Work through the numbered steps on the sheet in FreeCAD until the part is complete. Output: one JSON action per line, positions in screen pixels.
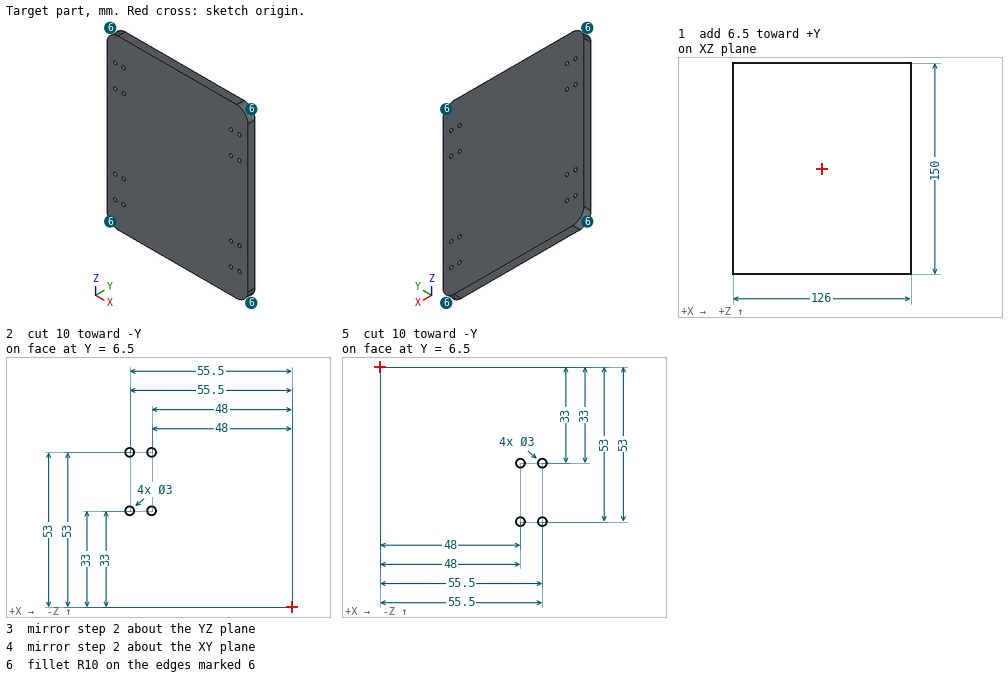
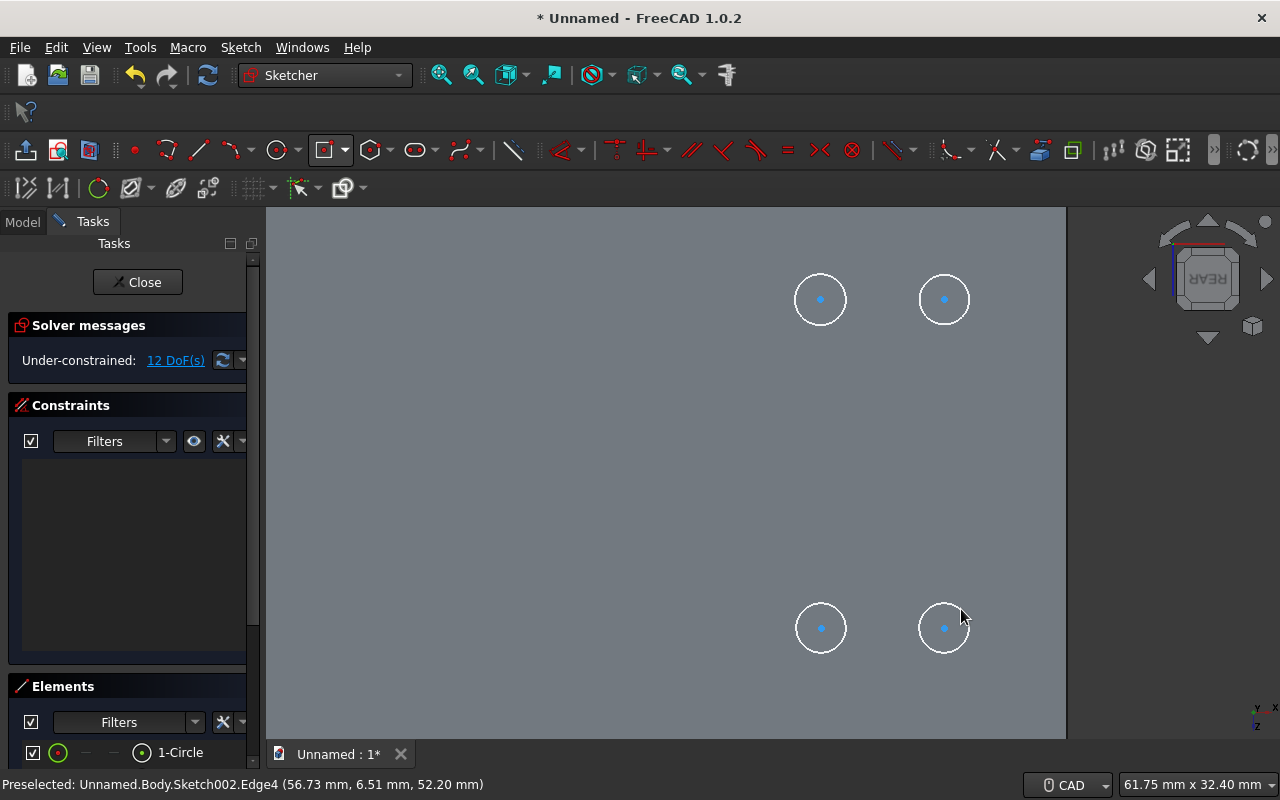
{"action": "left_click", "coordinate": [962, 282]}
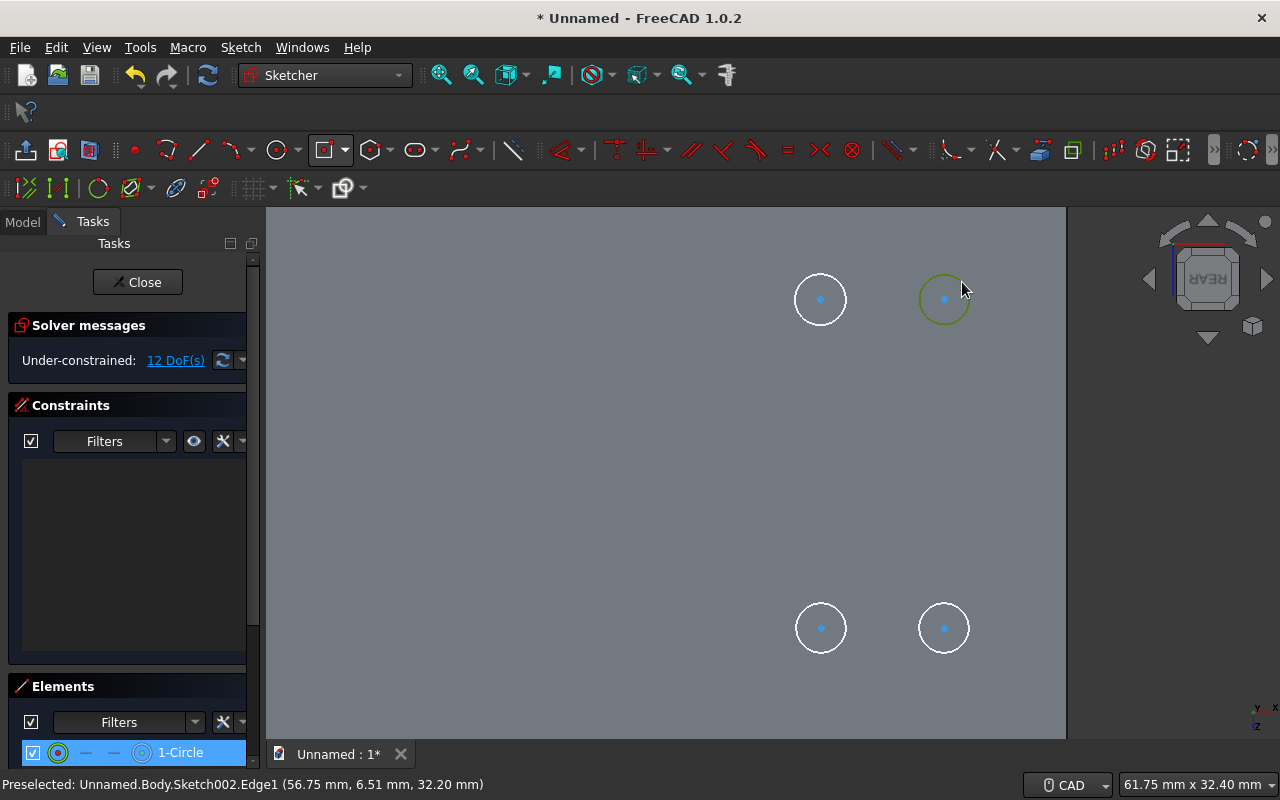
{"action": "left_click", "coordinate": [838, 282]}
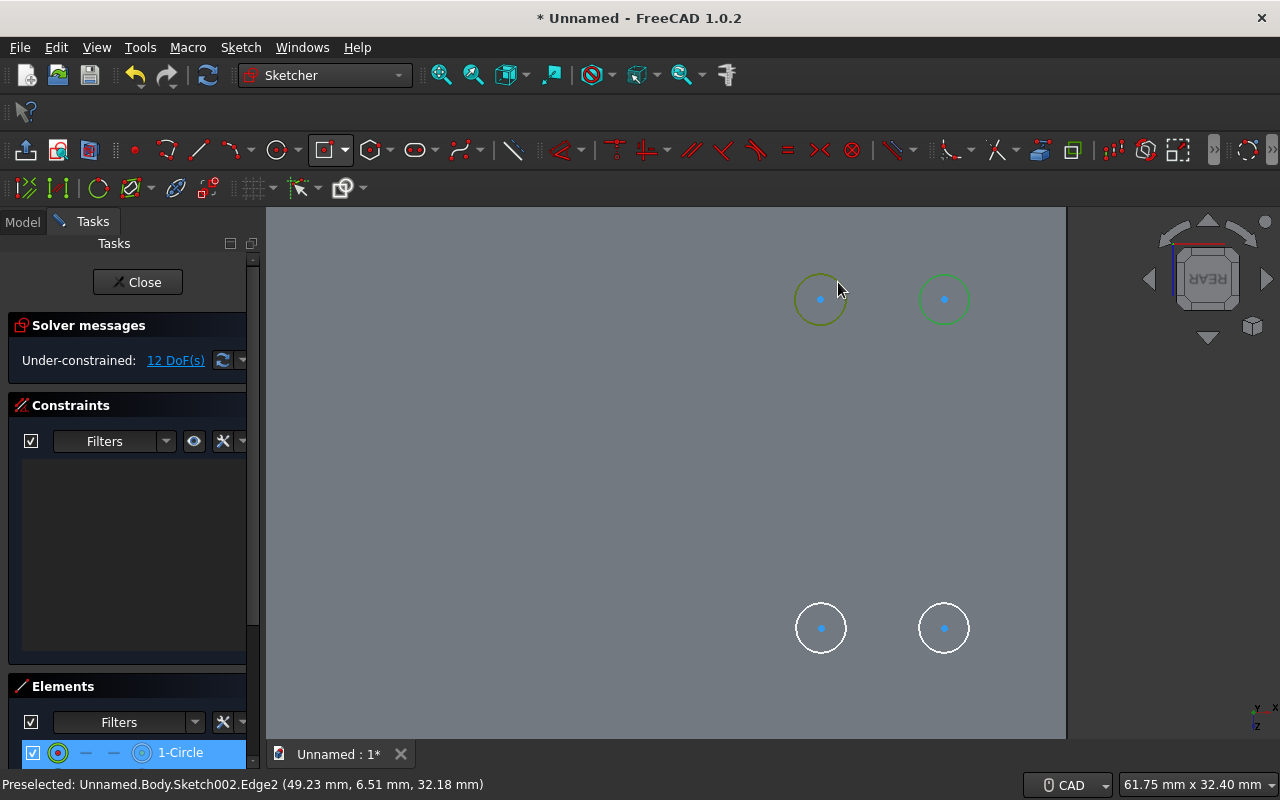
{"action": "left_click", "coordinate": [838, 610]}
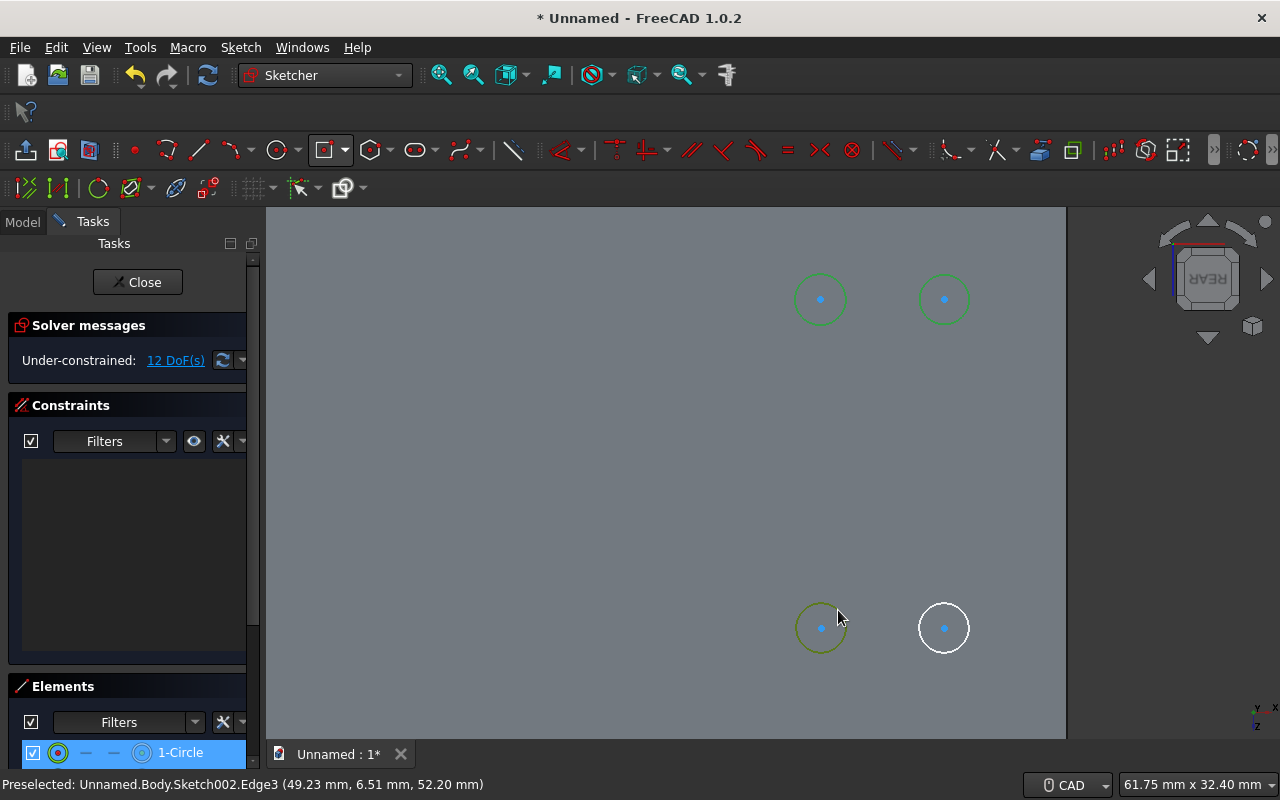
{"action": "left_click", "coordinate": [961, 610]}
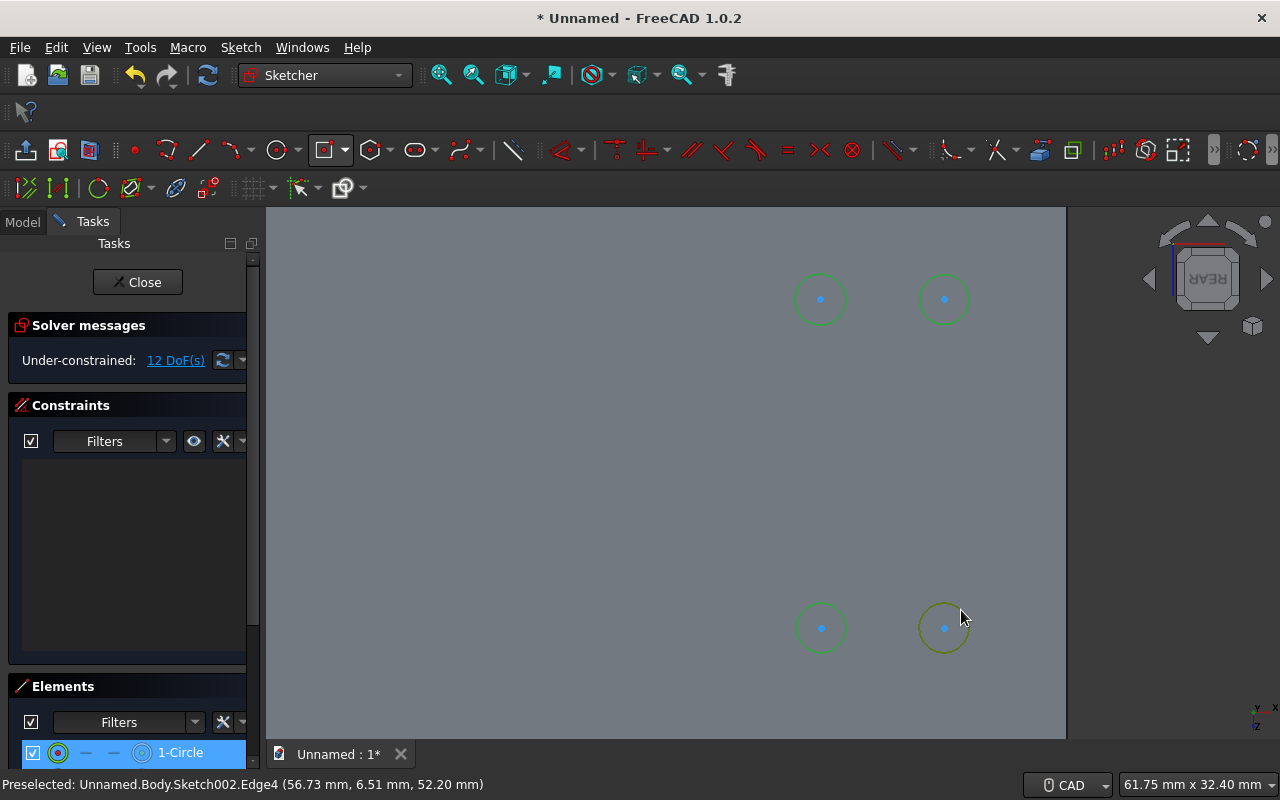
{"action": "left_click", "coordinate": [788, 150]}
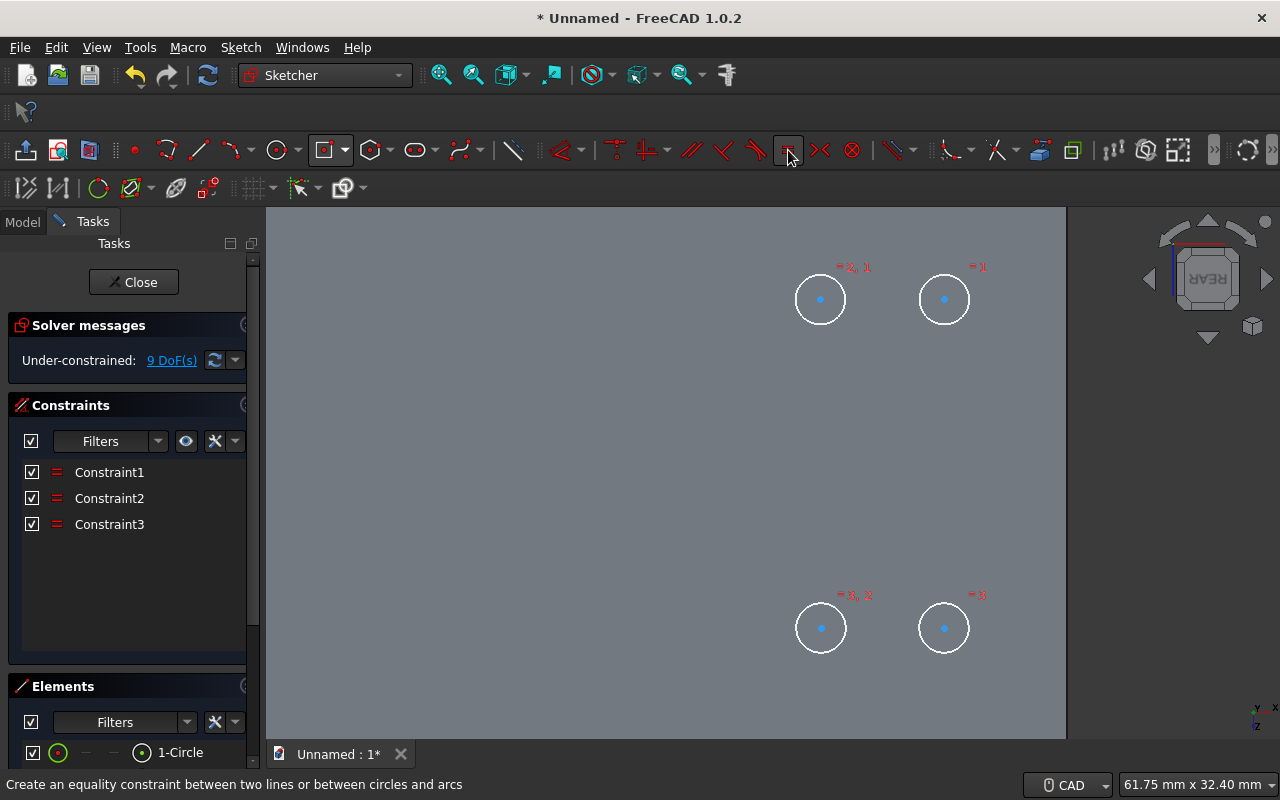
{"action": "left_click", "coordinate": [560, 150]}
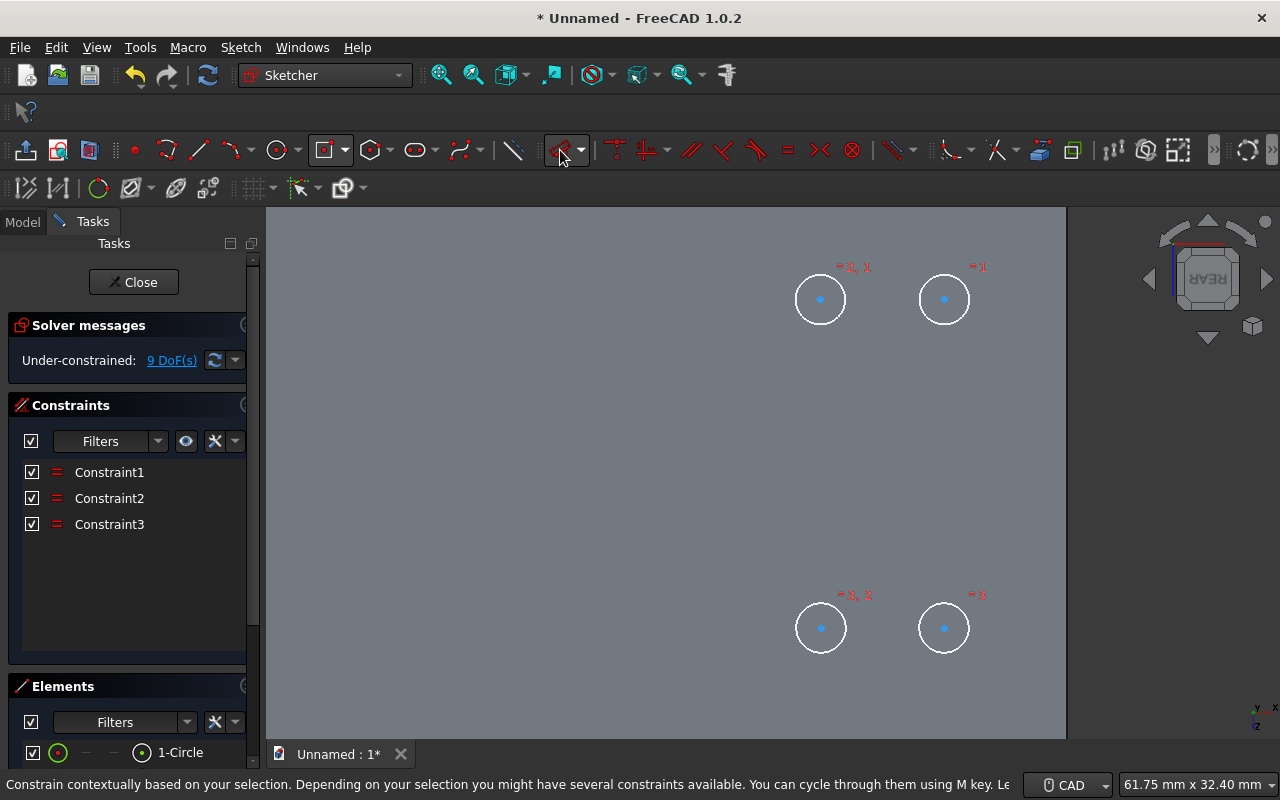
{"action": "left_click", "coordinate": [962, 282]}
{"action": "left_click", "coordinate": [985, 259]}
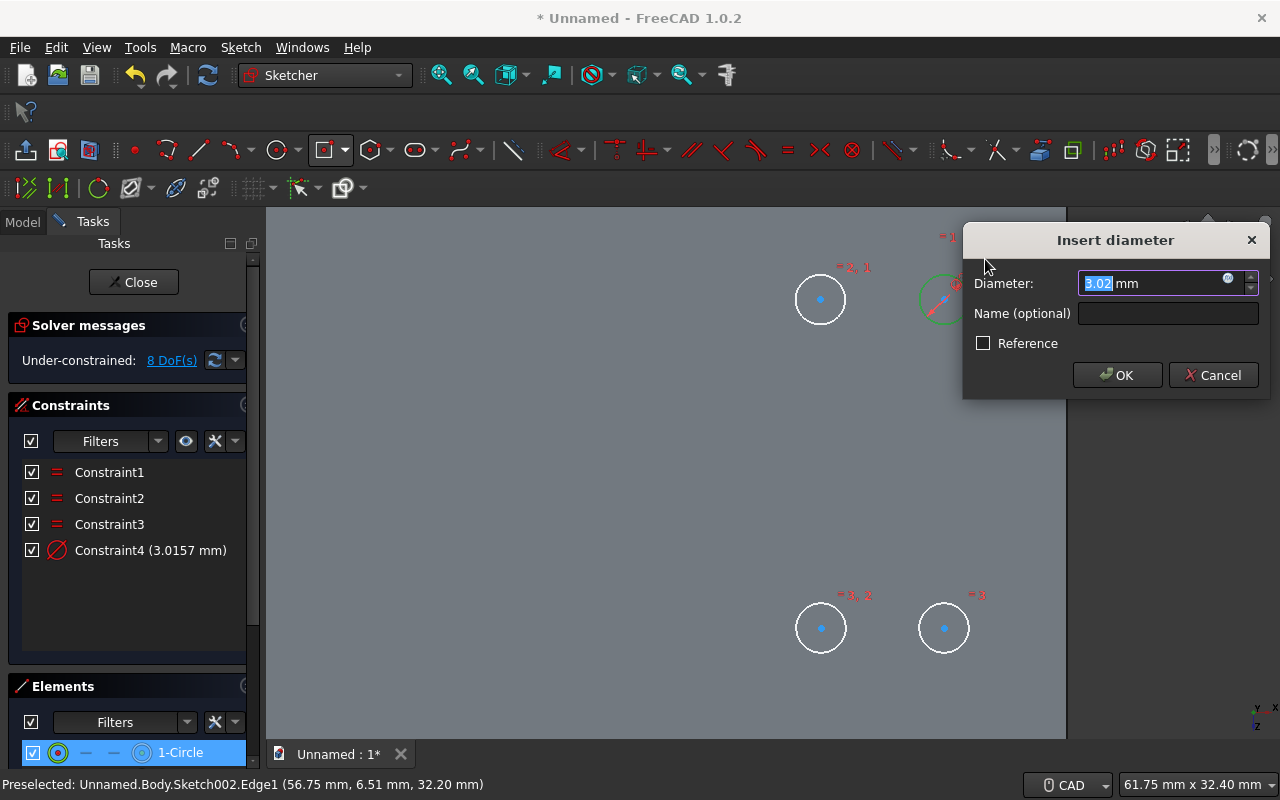
{"action": "type", "text": "3"}
{"action": "key", "text": "Return"}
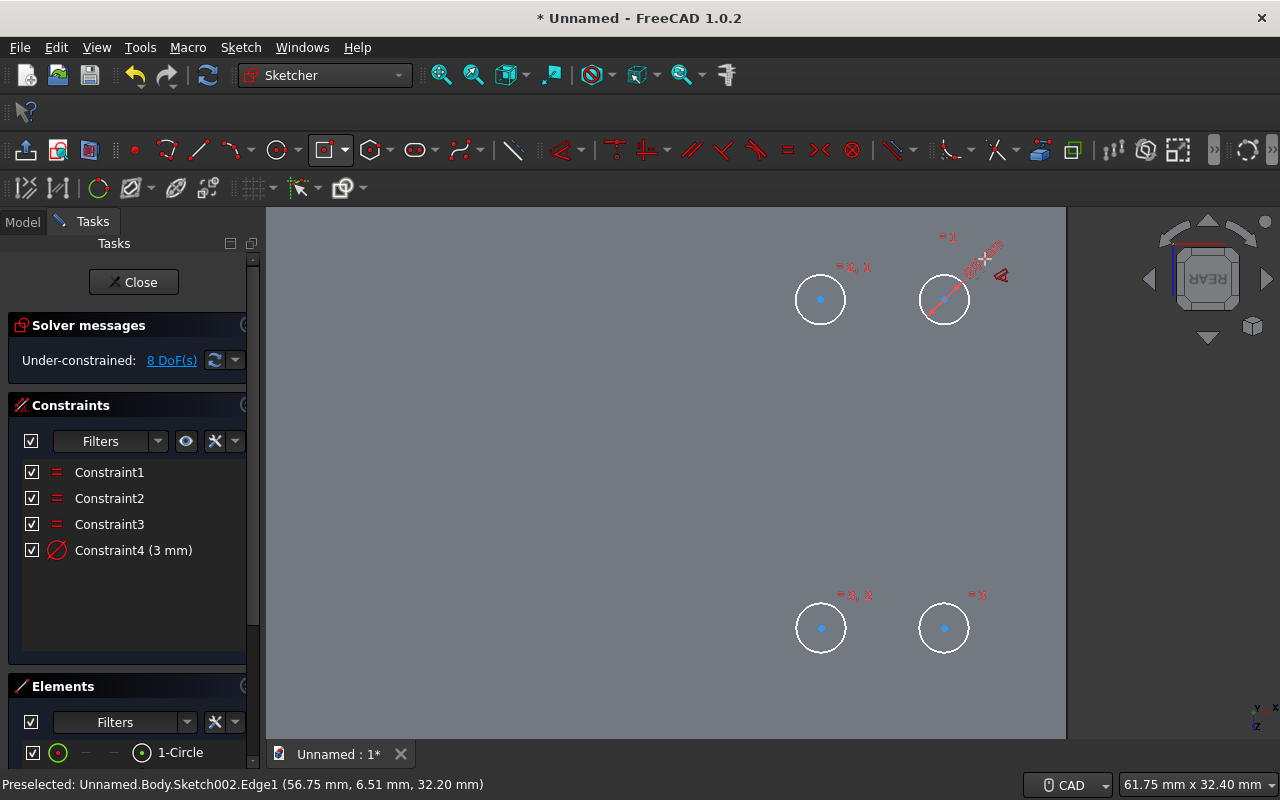
{"action": "left_click", "coordinate": [944, 300]}
{"action": "left_click", "coordinate": [978, 282]}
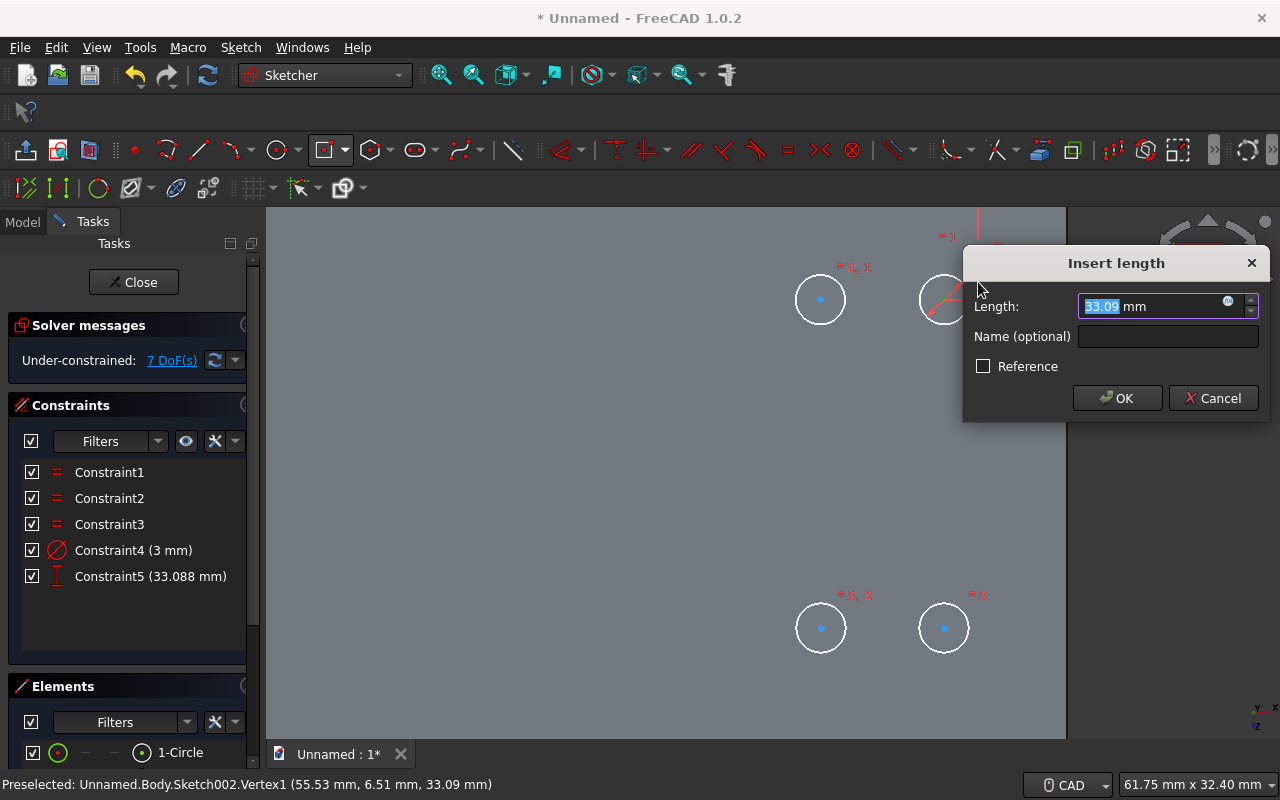
{"action": "type", "text": "33"}
{"action": "key", "text": "Return"}